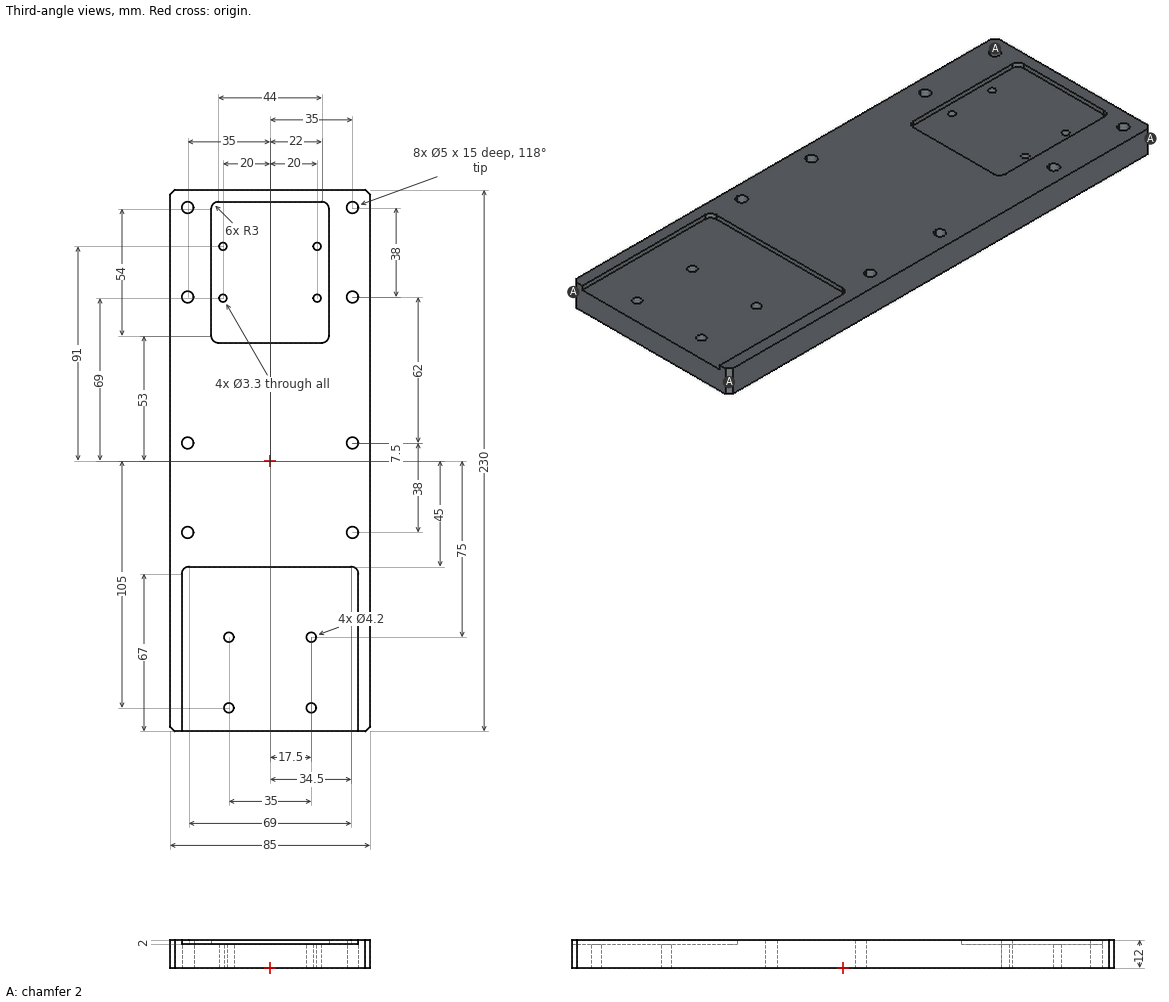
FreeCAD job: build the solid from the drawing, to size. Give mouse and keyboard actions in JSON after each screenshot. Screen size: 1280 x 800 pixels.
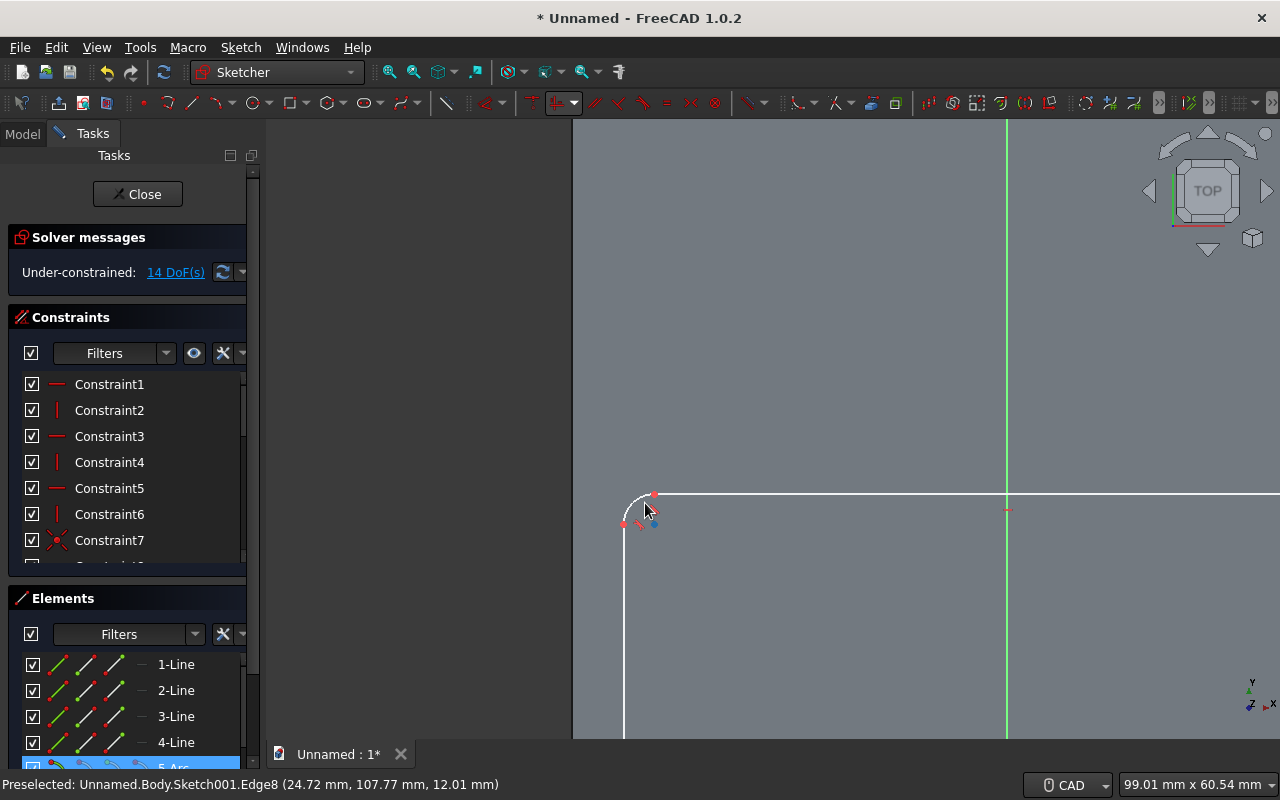
{"action": "left_click", "coordinate": [640, 498]}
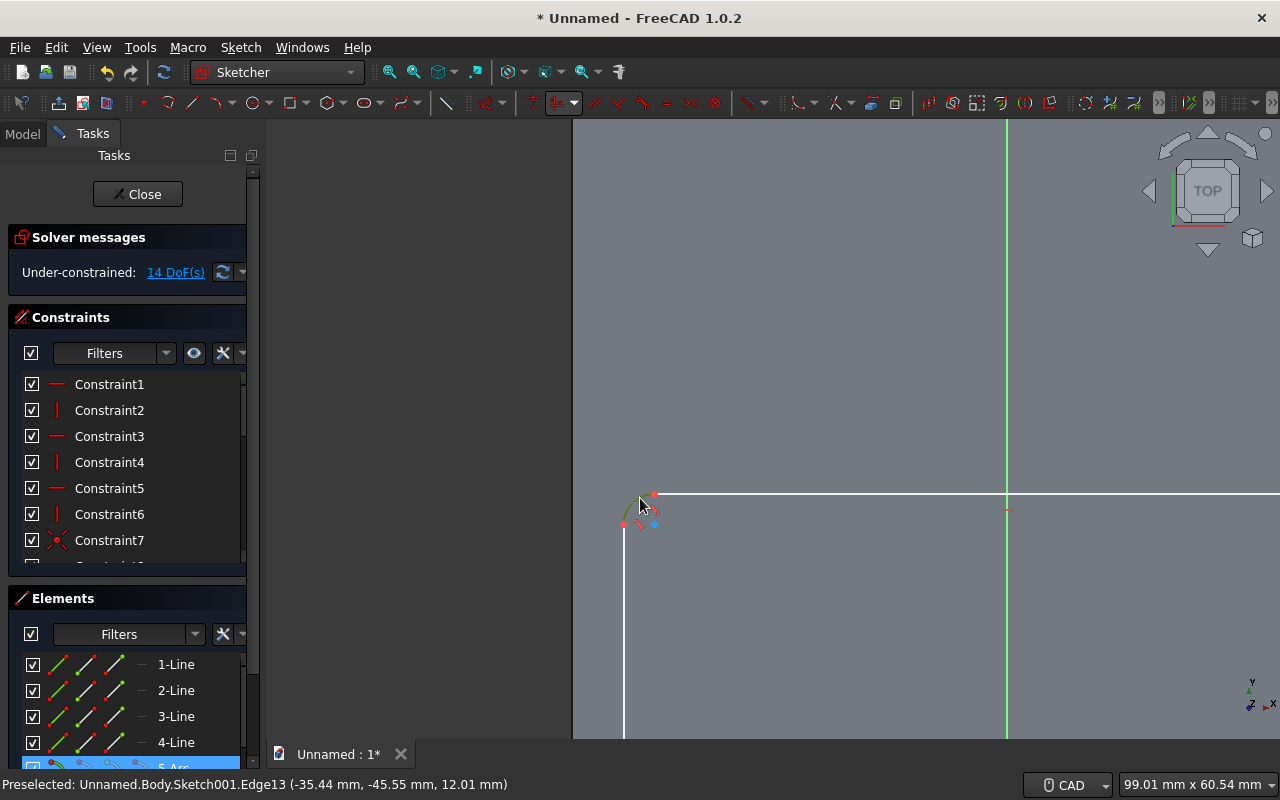
{"action": "scroll", "coordinate": [645, 503], "scroll_direction": "down", "scroll_amount": 9}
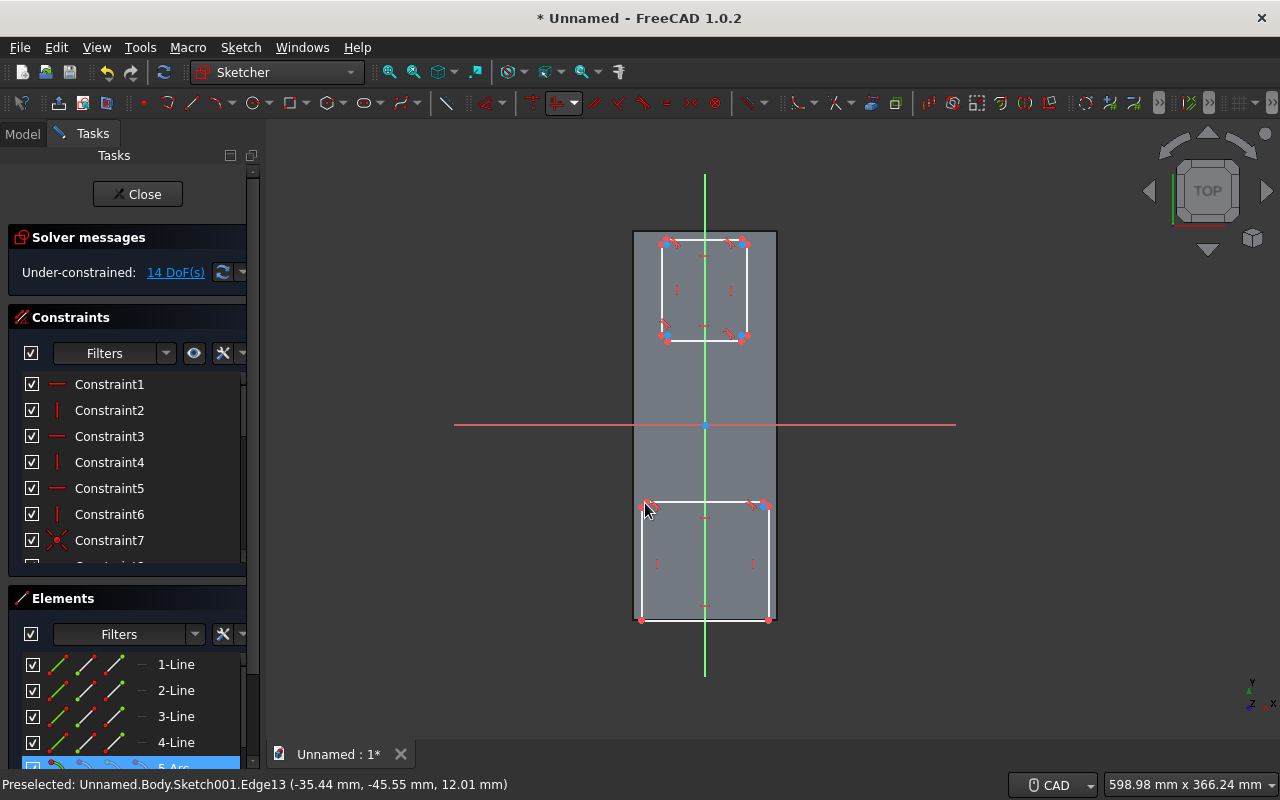
{"action": "scroll", "coordinate": [768, 505], "scroll_direction": "up", "scroll_amount": 10}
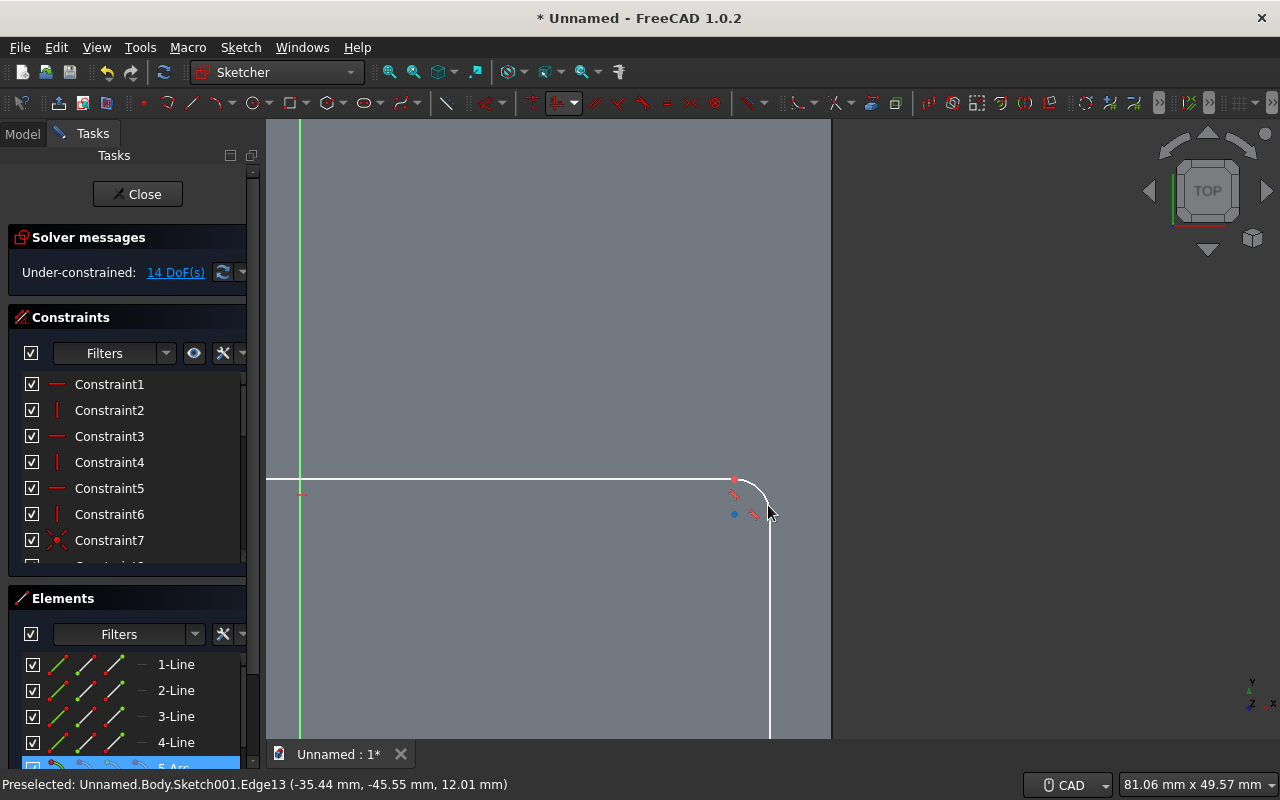
{"action": "left_click", "coordinate": [766, 498]}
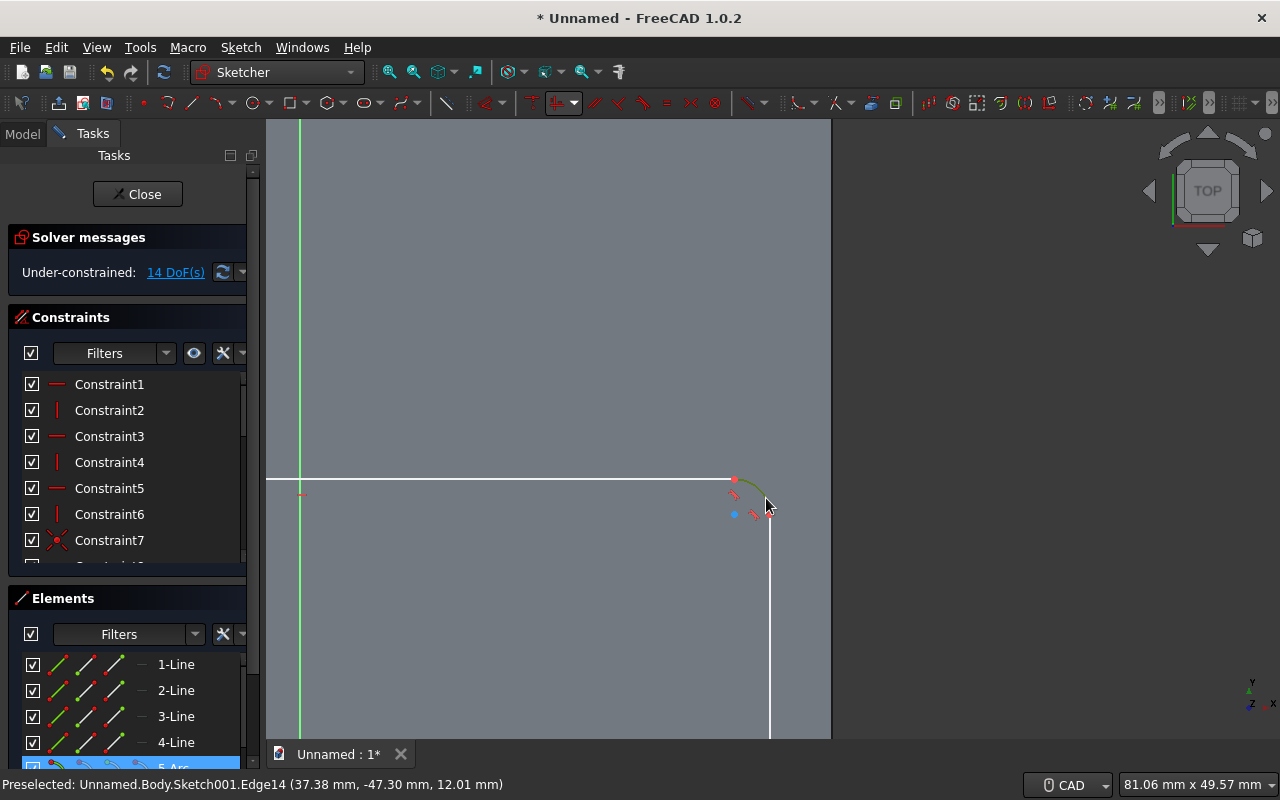
{"action": "left_click", "coordinate": [668, 104]}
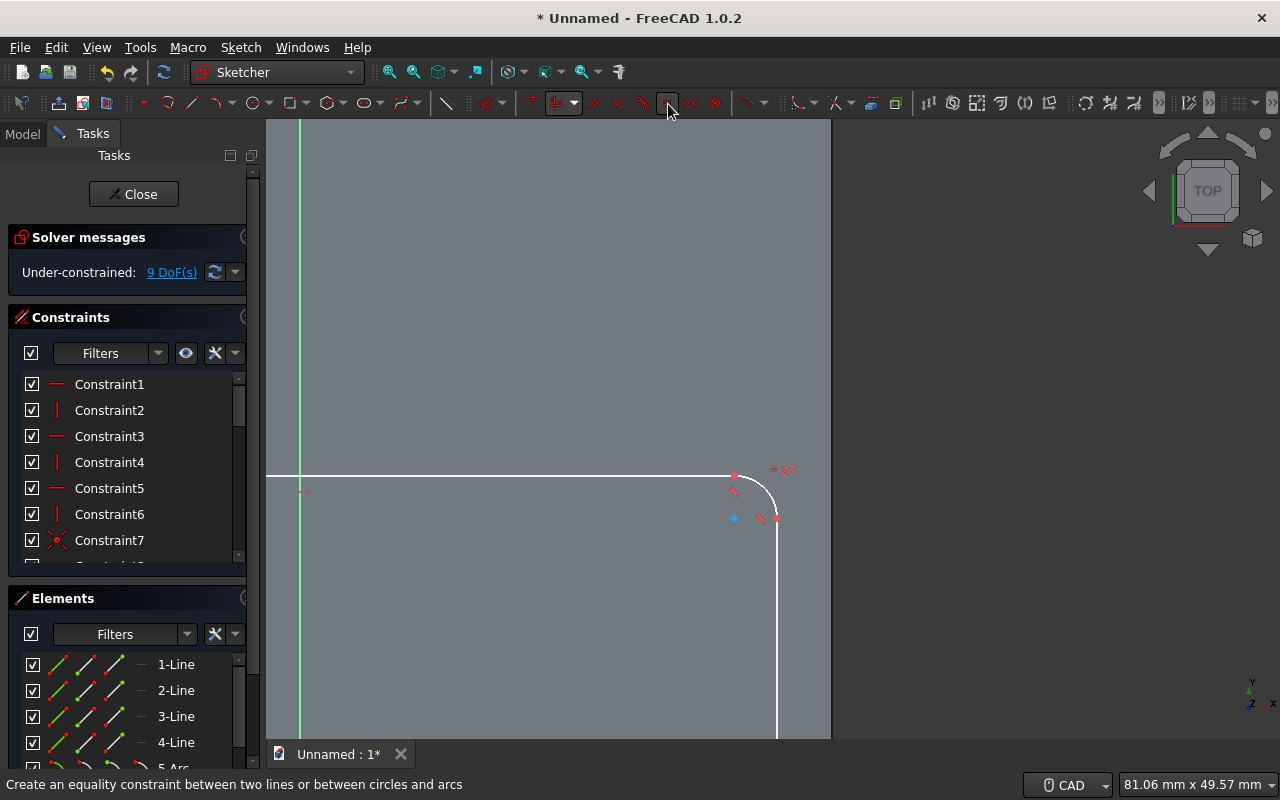
{"action": "scroll", "coordinate": [768, 505], "scroll_direction": "down", "scroll_amount": 10}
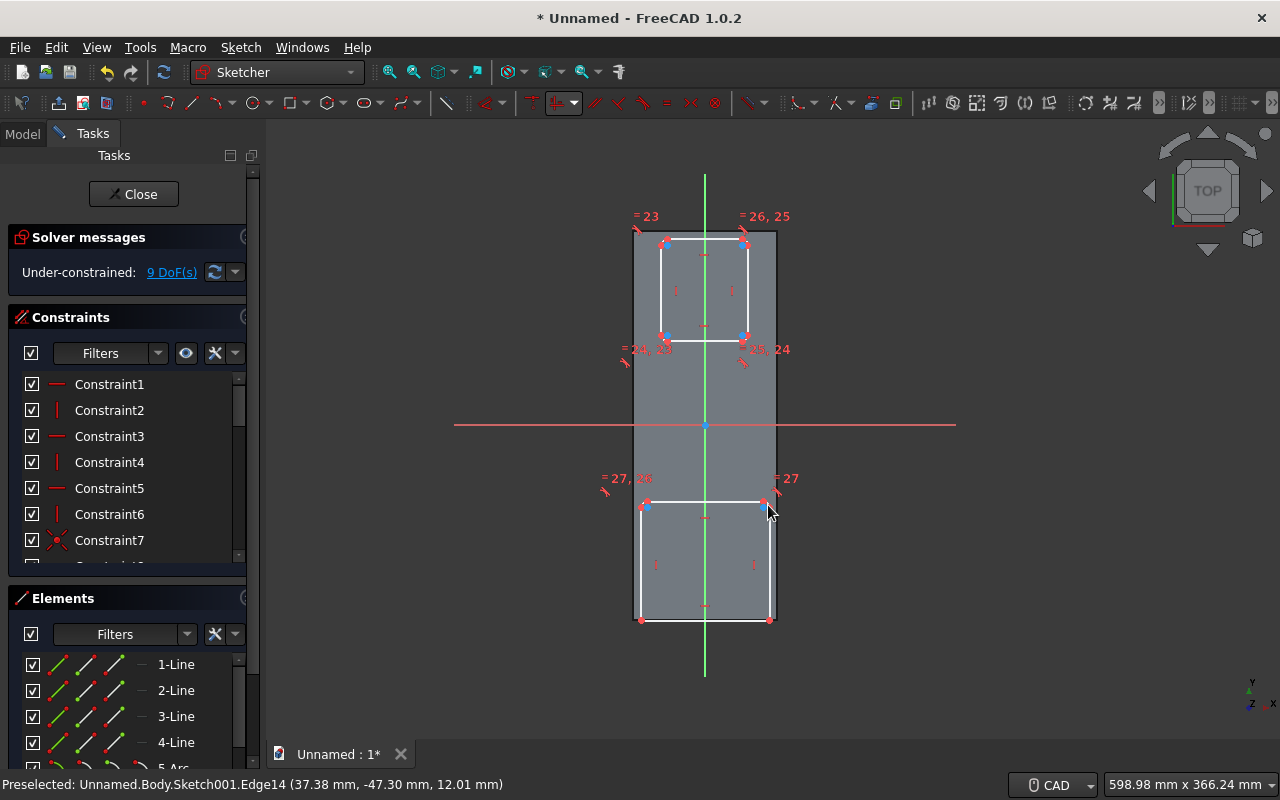
{"action": "scroll", "coordinate": [664, 240], "scroll_direction": "up", "scroll_amount": 11}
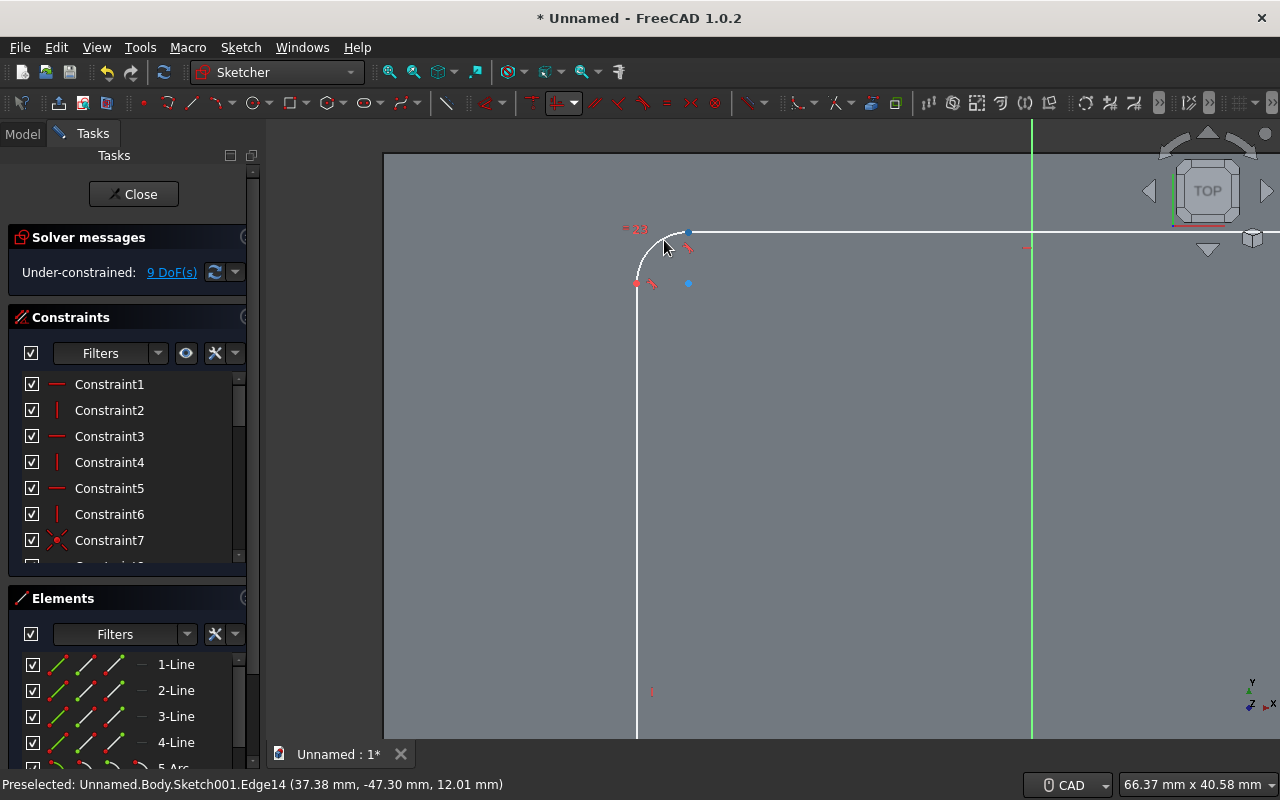
{"action": "left_click", "coordinate": [665, 238]}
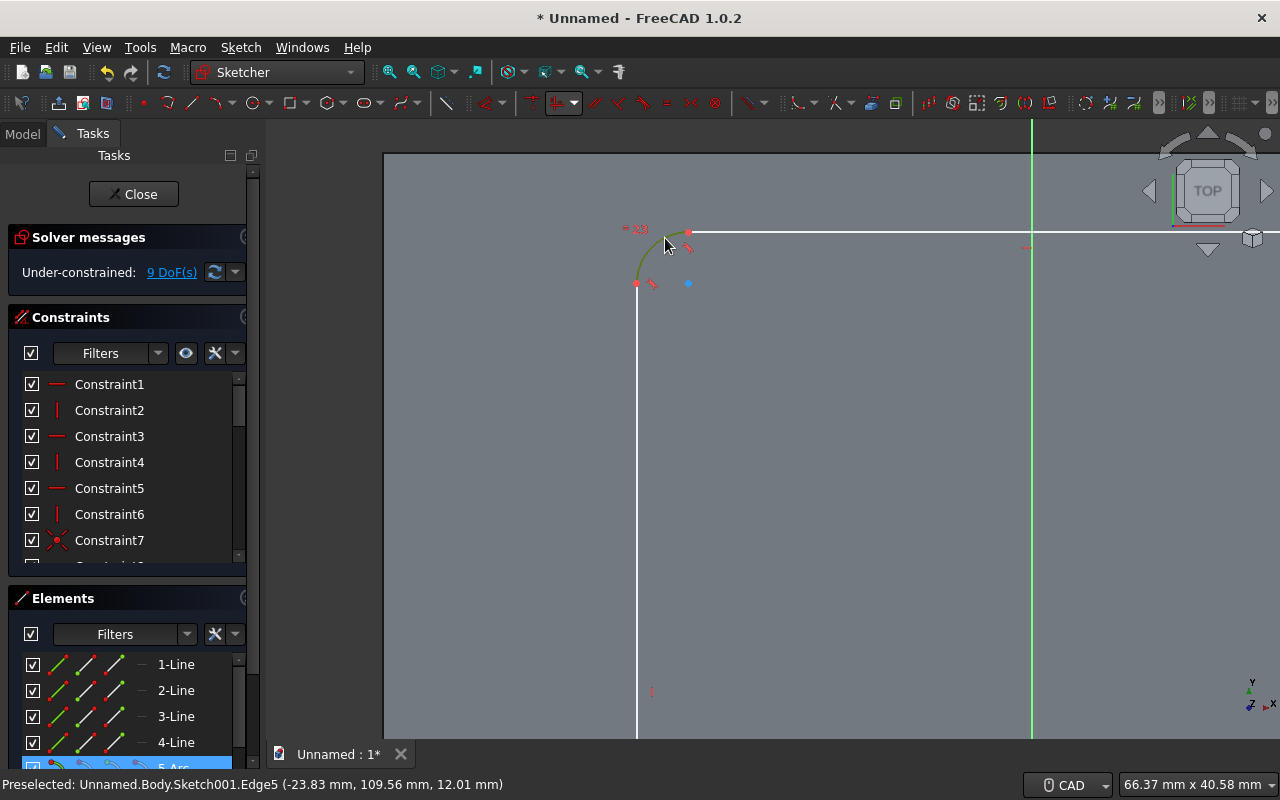
{"action": "key", "text": "k r"}